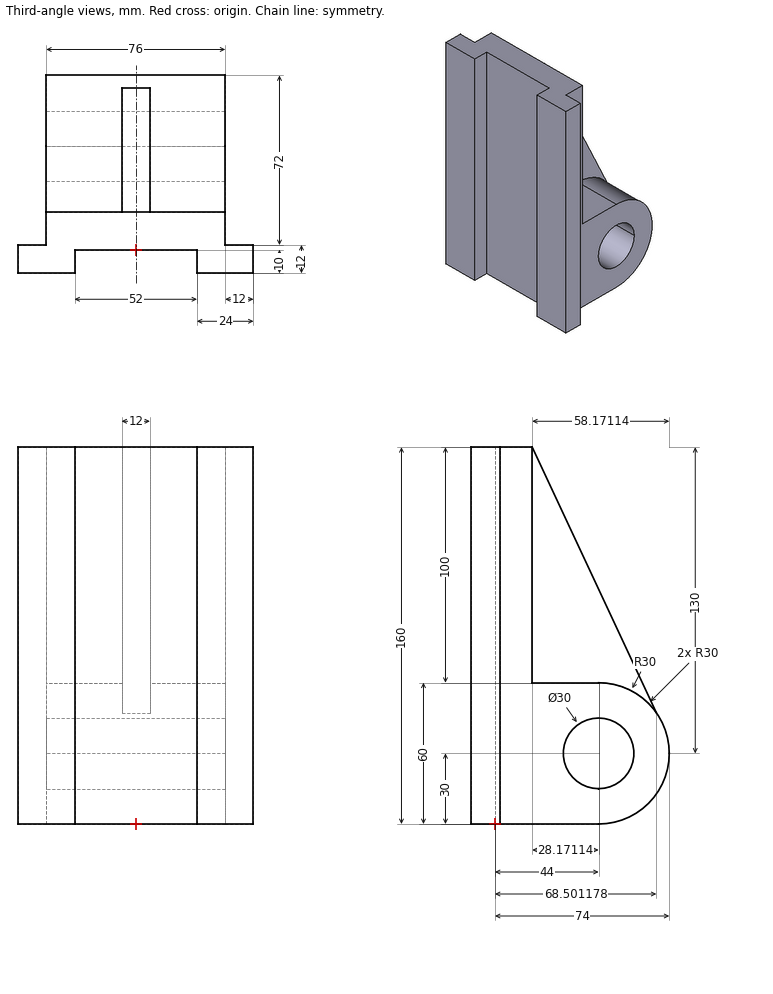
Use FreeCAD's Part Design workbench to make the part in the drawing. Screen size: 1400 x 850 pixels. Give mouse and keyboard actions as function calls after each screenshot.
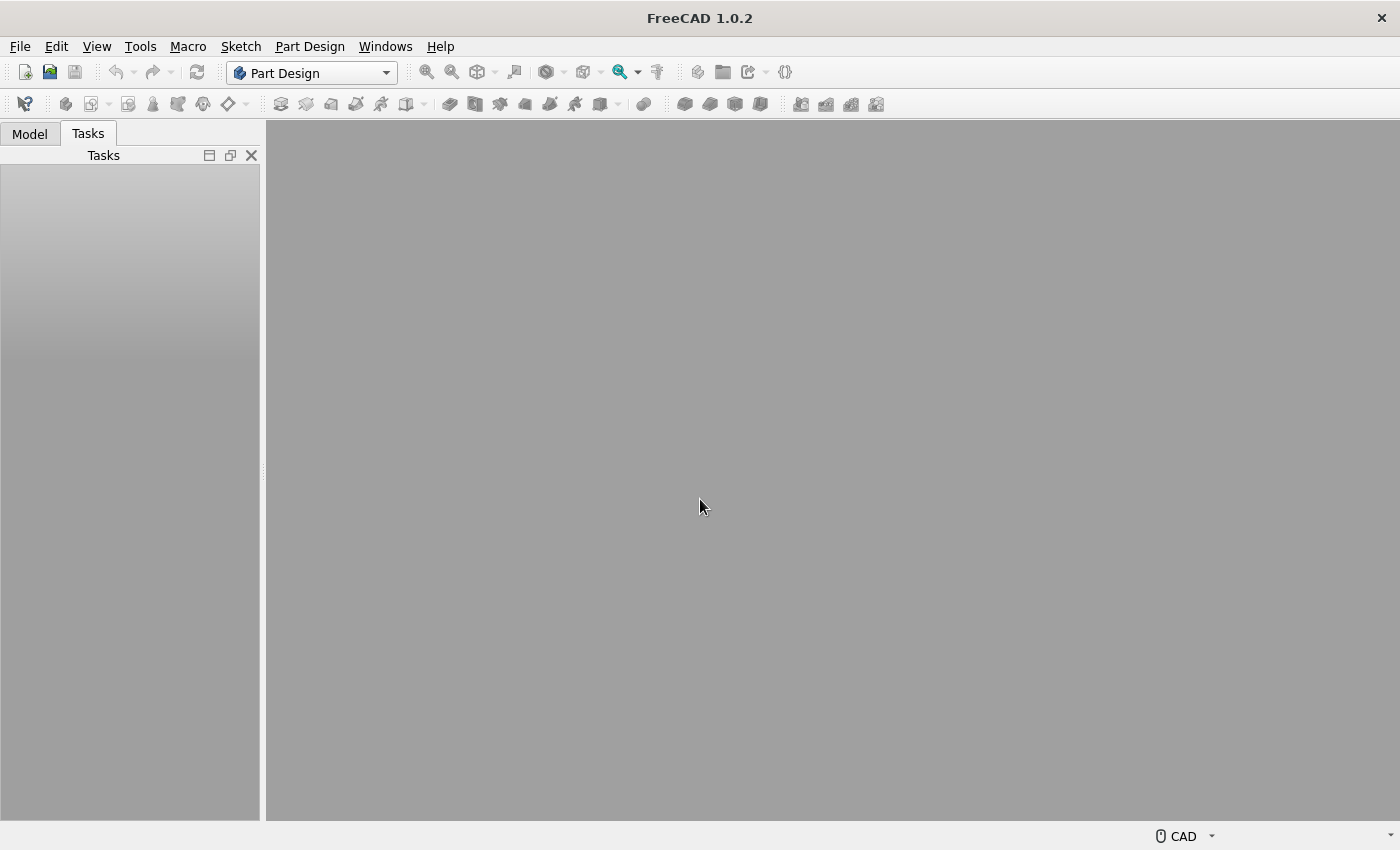
key(ctrl+n)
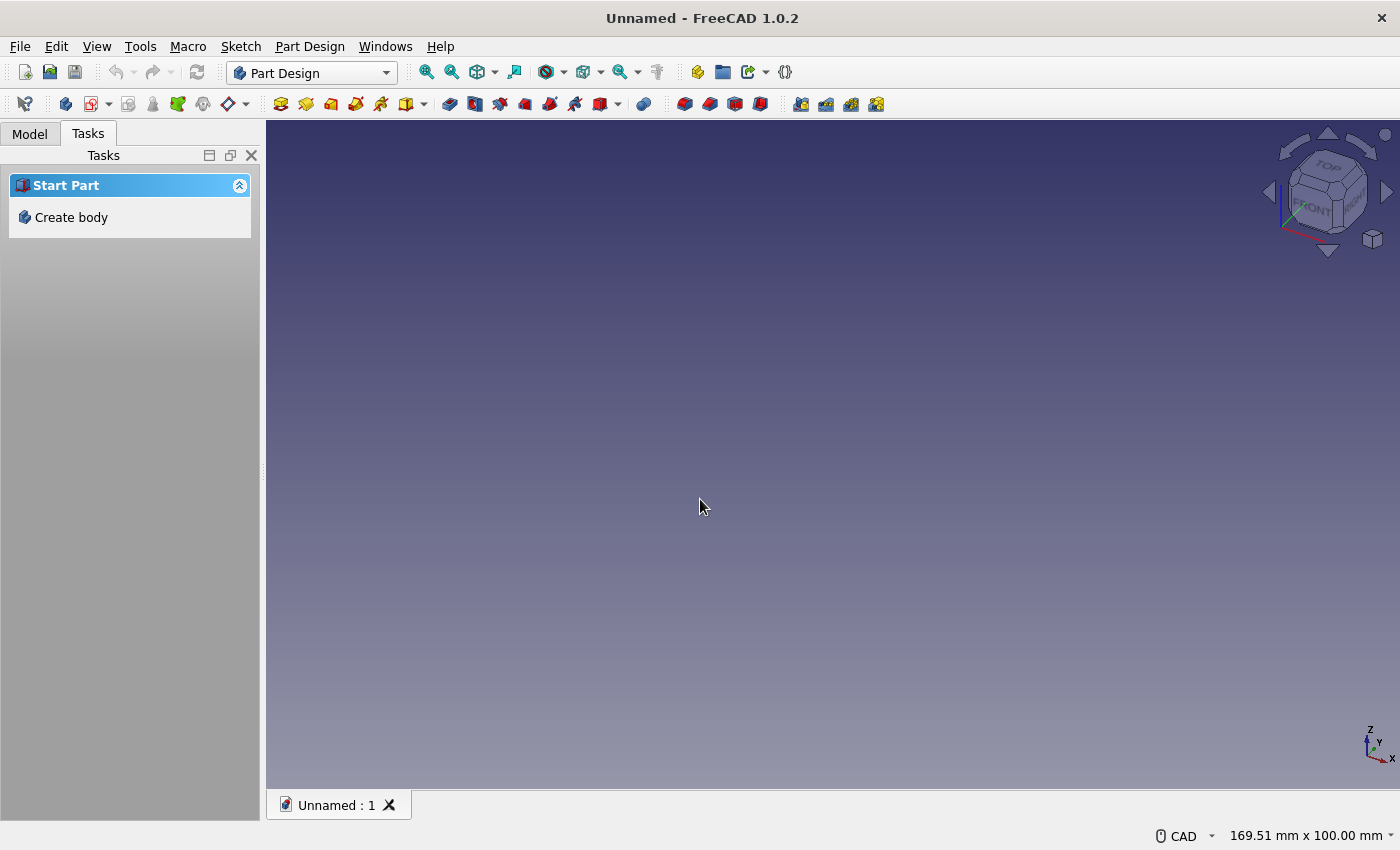
click(90, 104)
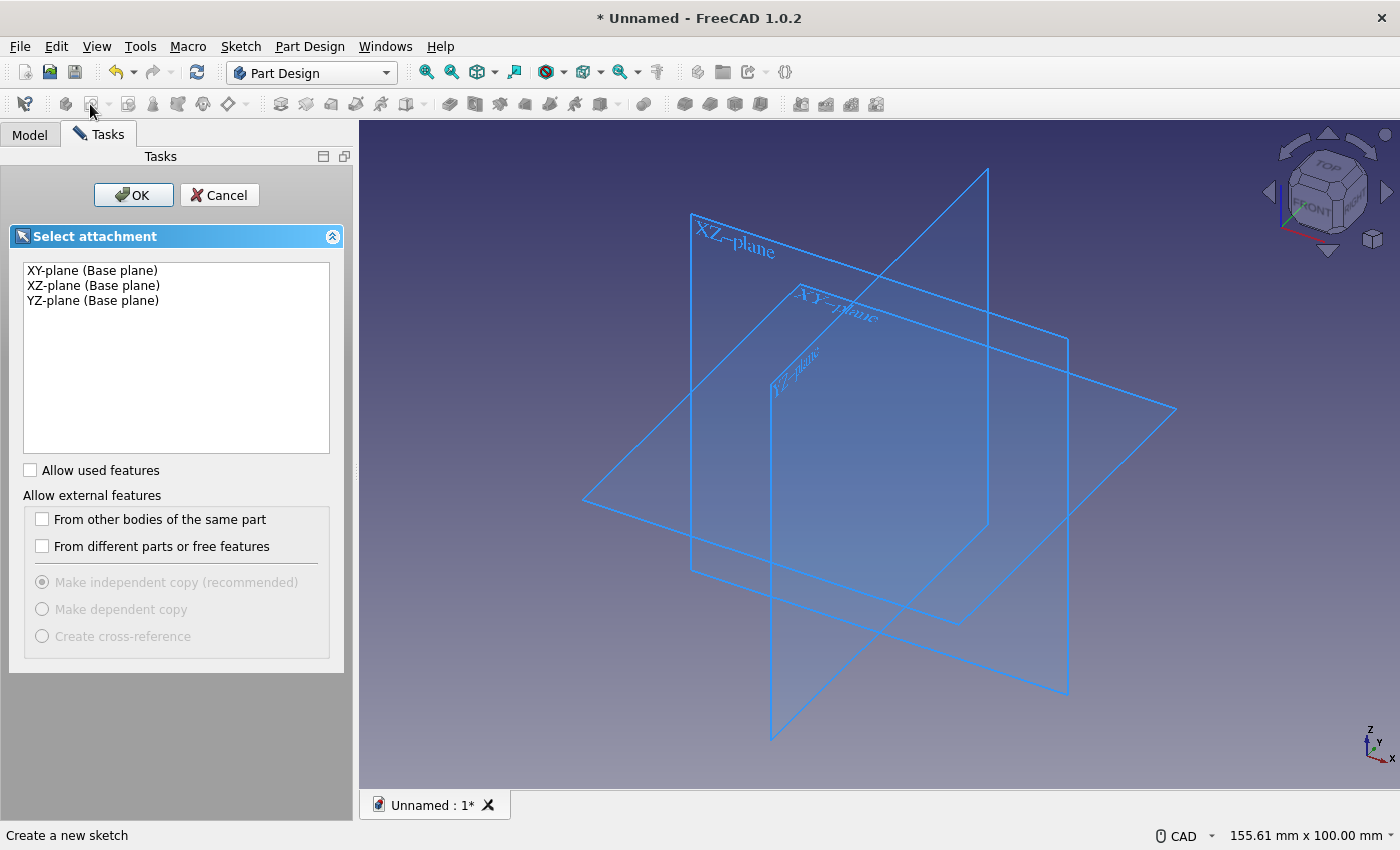
click(84, 270)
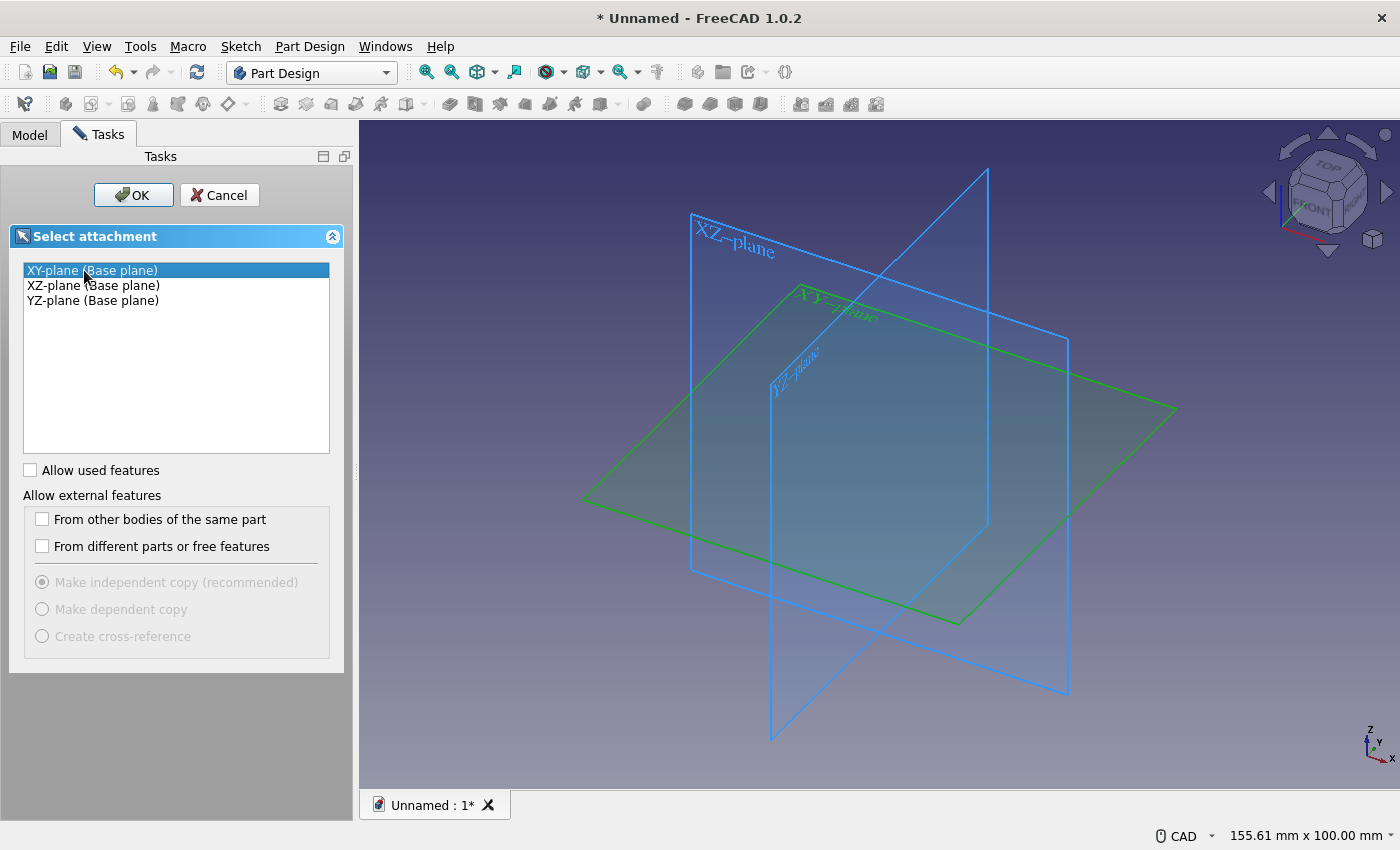
click(134, 195)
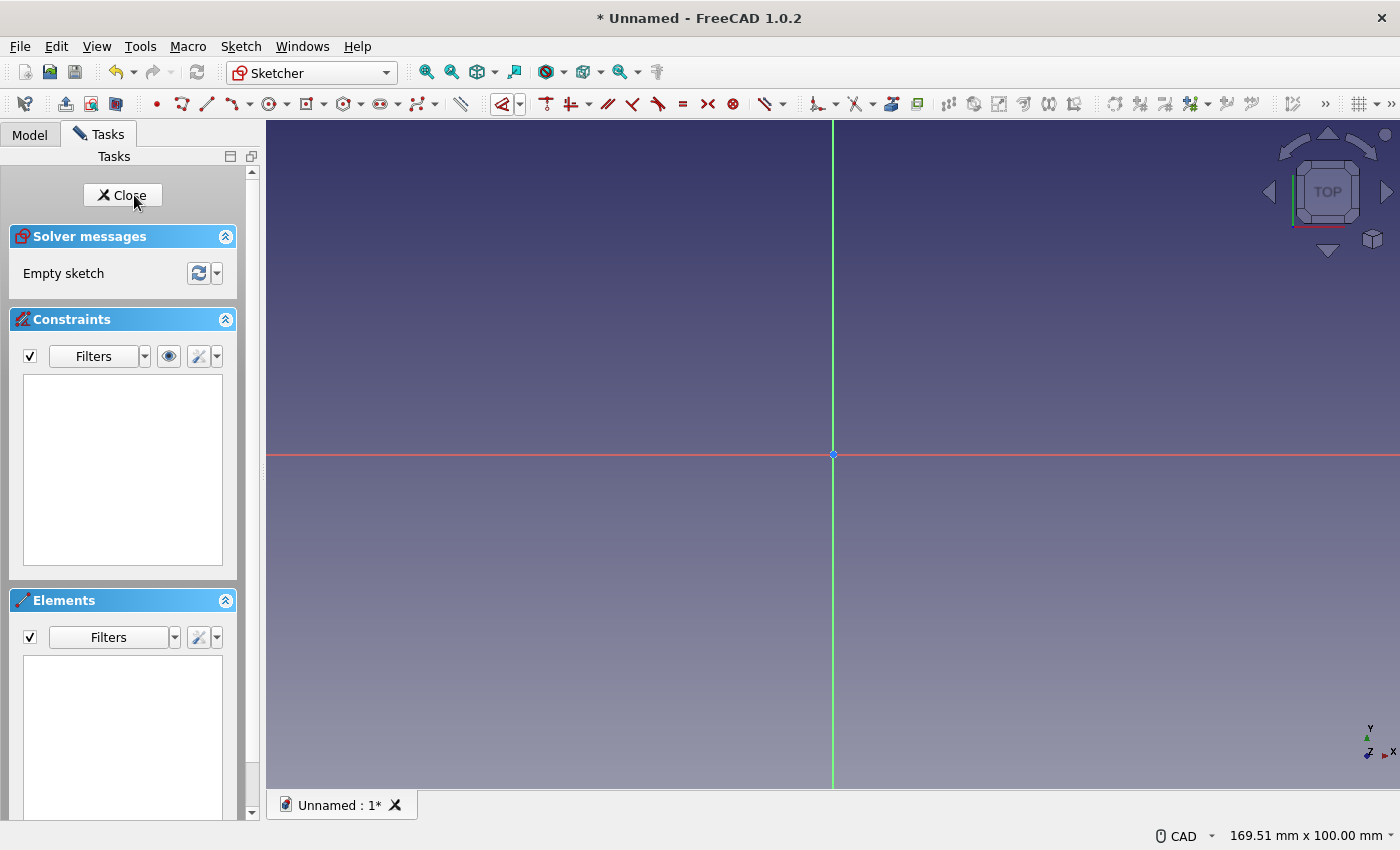
scroll(625, 761, down, 2)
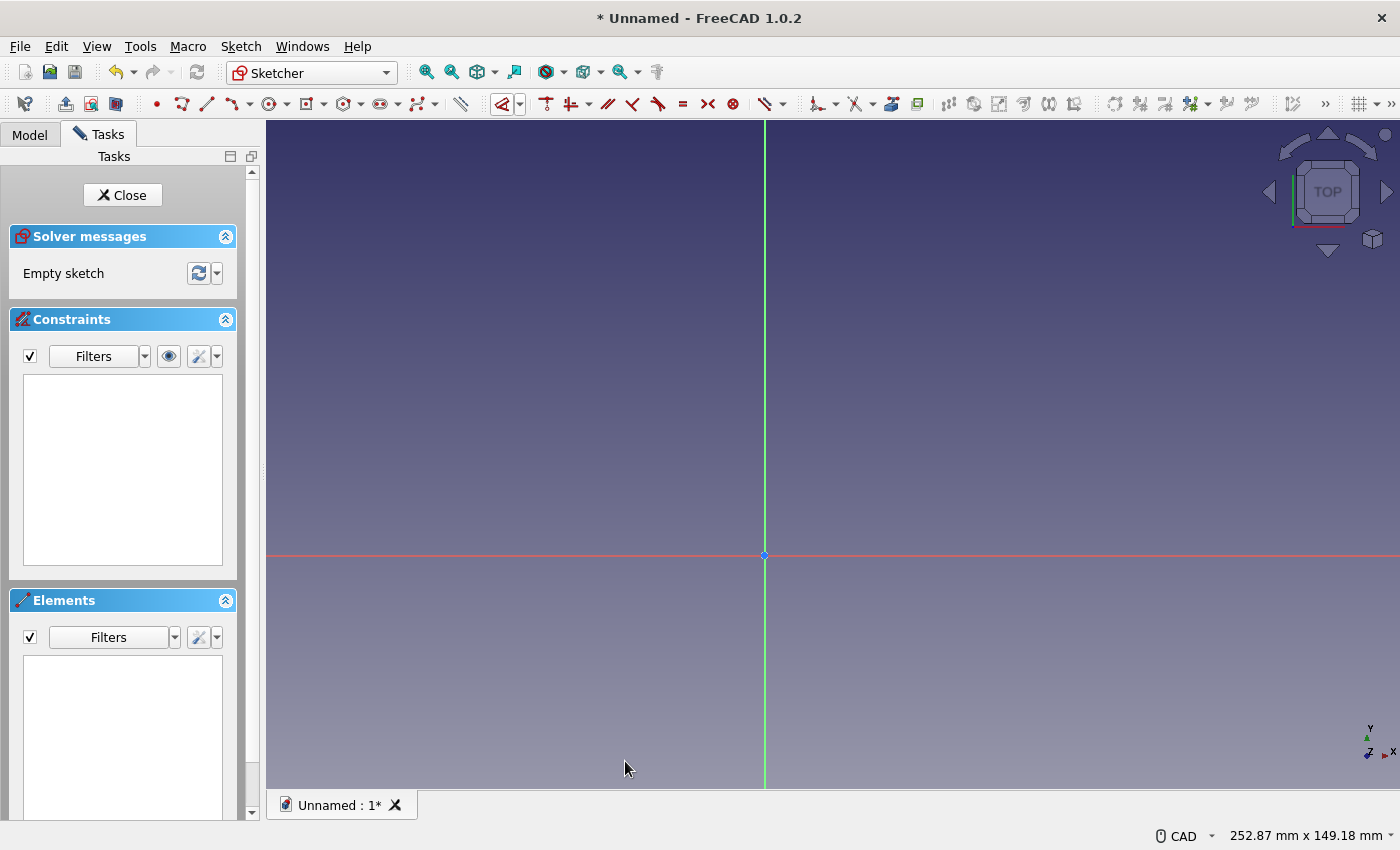
click(182, 104)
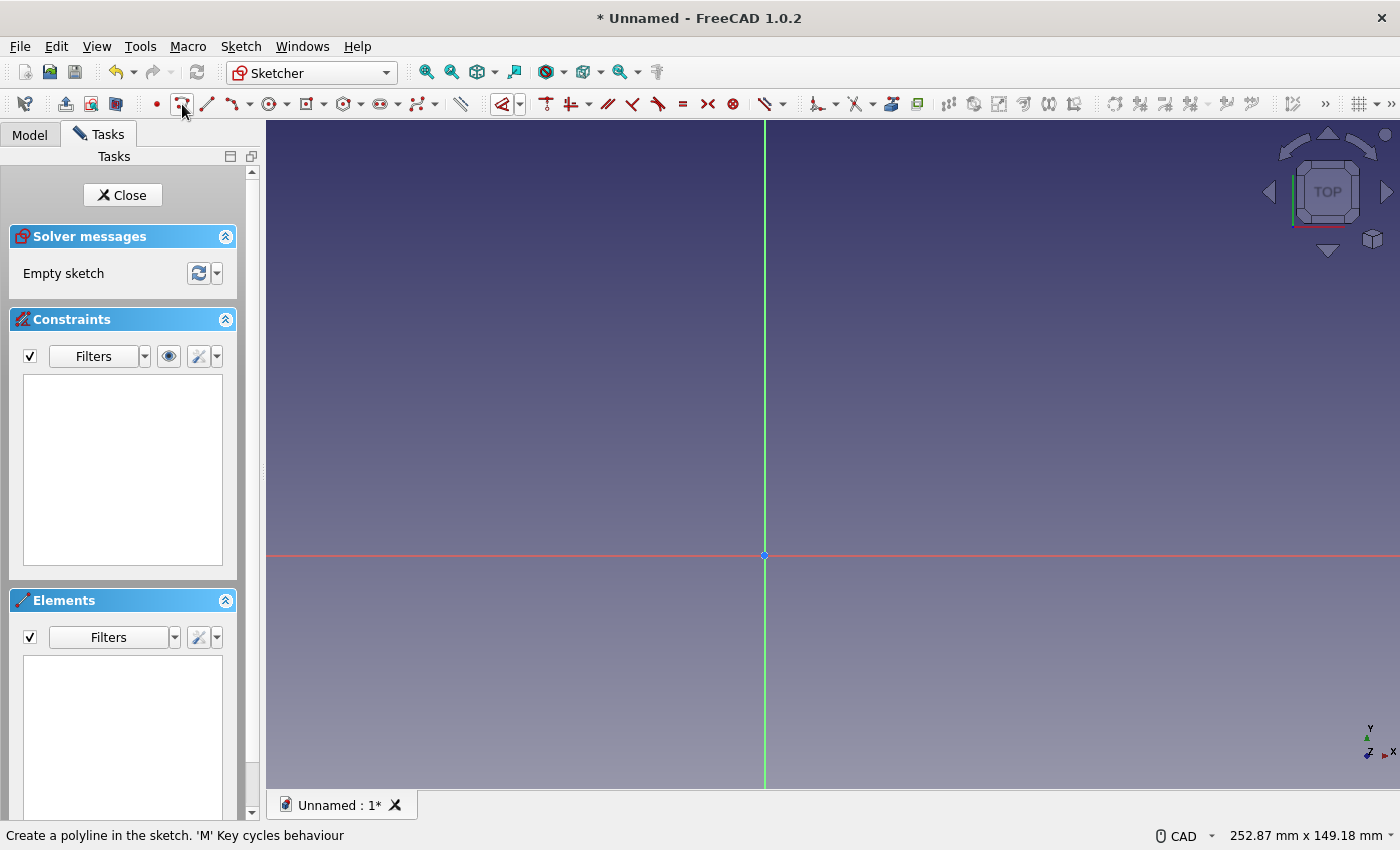
click(648, 556)
click(881, 547)
click(881, 601)
click(989, 601)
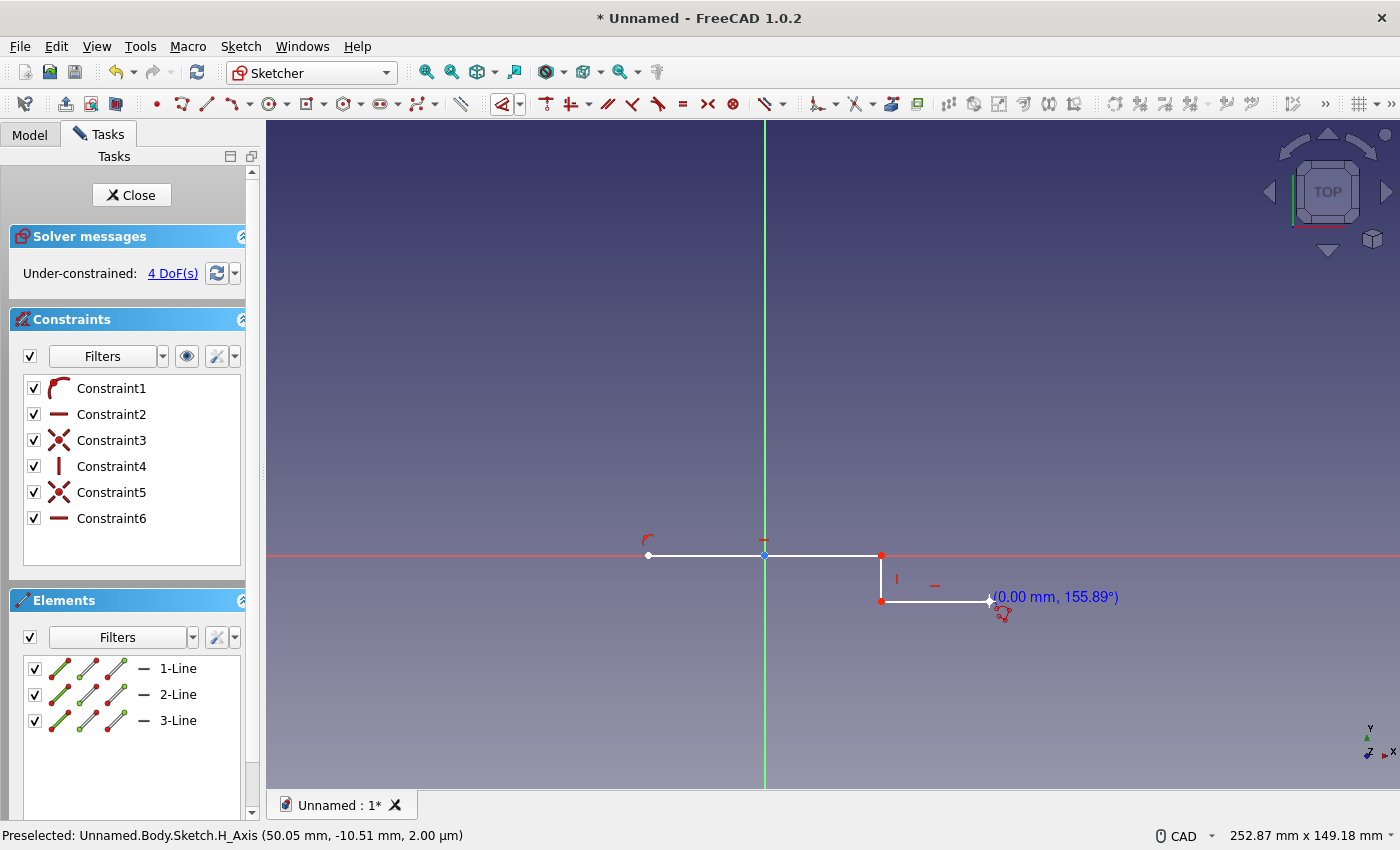
scroll(989, 547, up, 3)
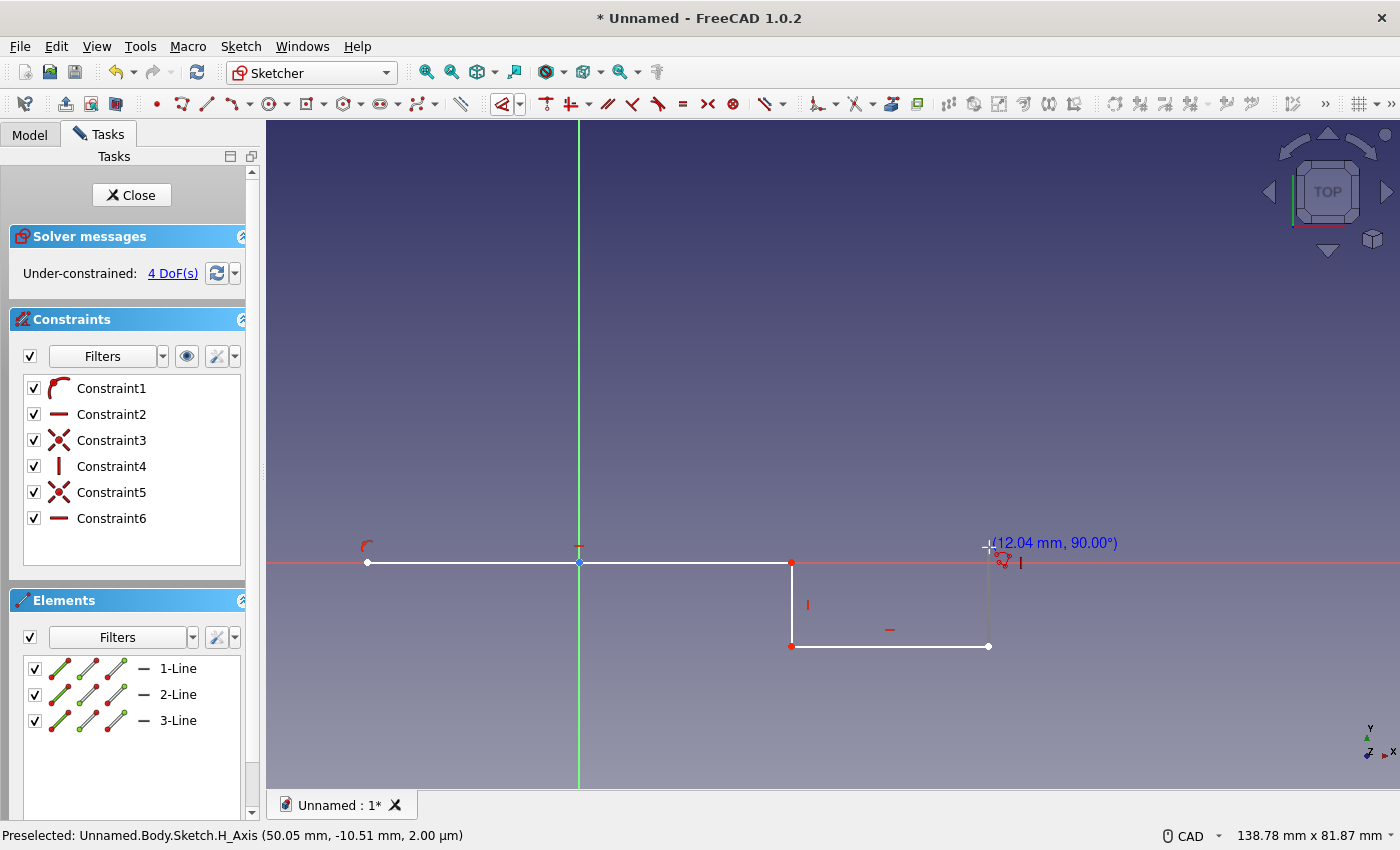
click(988, 546)
click(890, 546)